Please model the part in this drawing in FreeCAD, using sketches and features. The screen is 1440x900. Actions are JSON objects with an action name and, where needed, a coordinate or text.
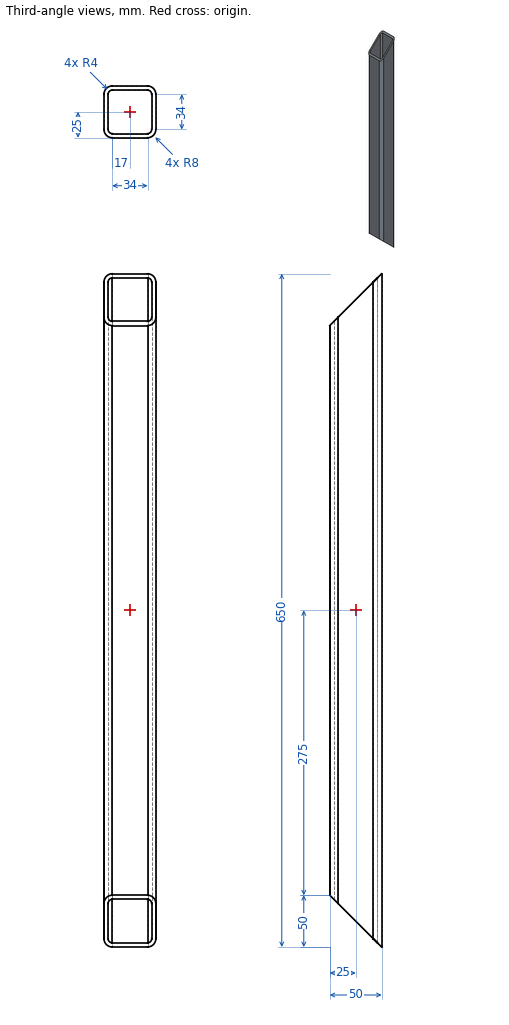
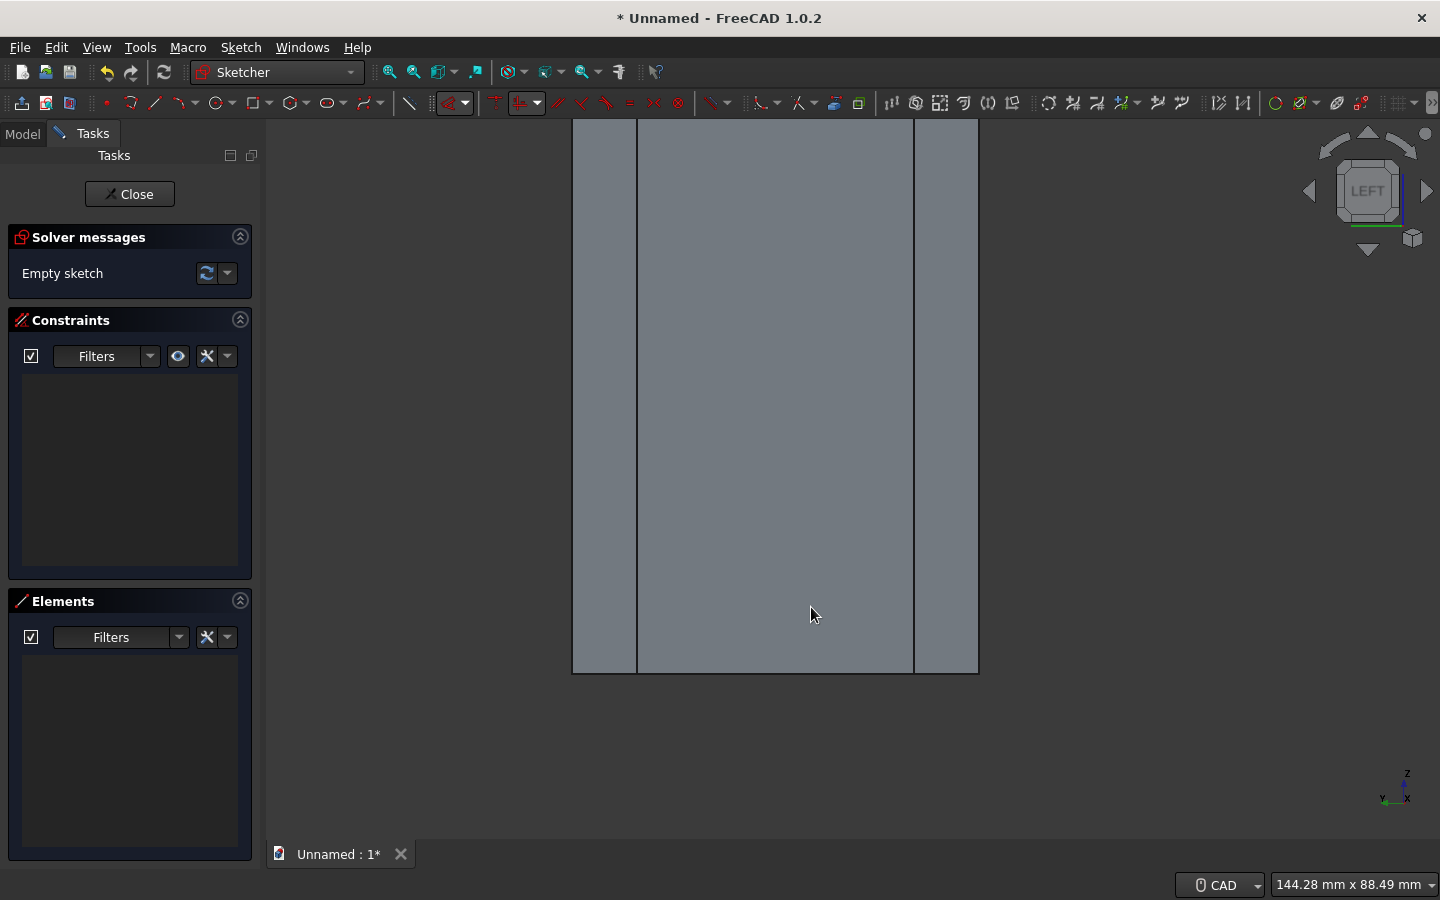
{"action": "left_click", "coordinate": [132, 104]}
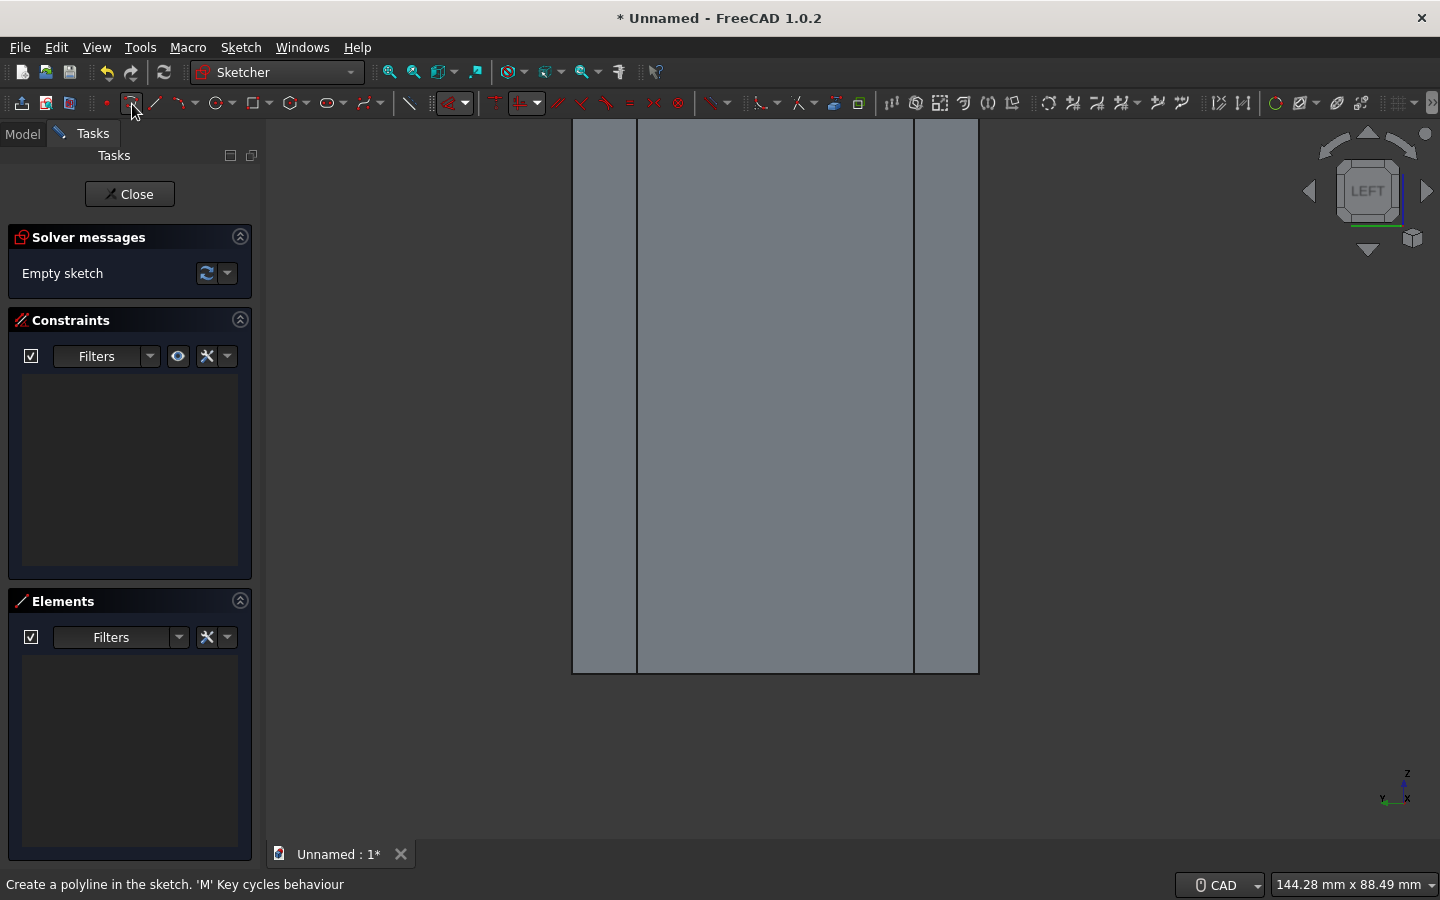
{"action": "left_click", "coordinate": [979, 267]}
{"action": "left_click", "coordinate": [572, 674]}
{"action": "left_click", "coordinate": [979, 674]}
{"action": "left_click", "coordinate": [979, 268]}
{"action": "key", "text": "Escape"}
{"action": "key", "text": "Escape"}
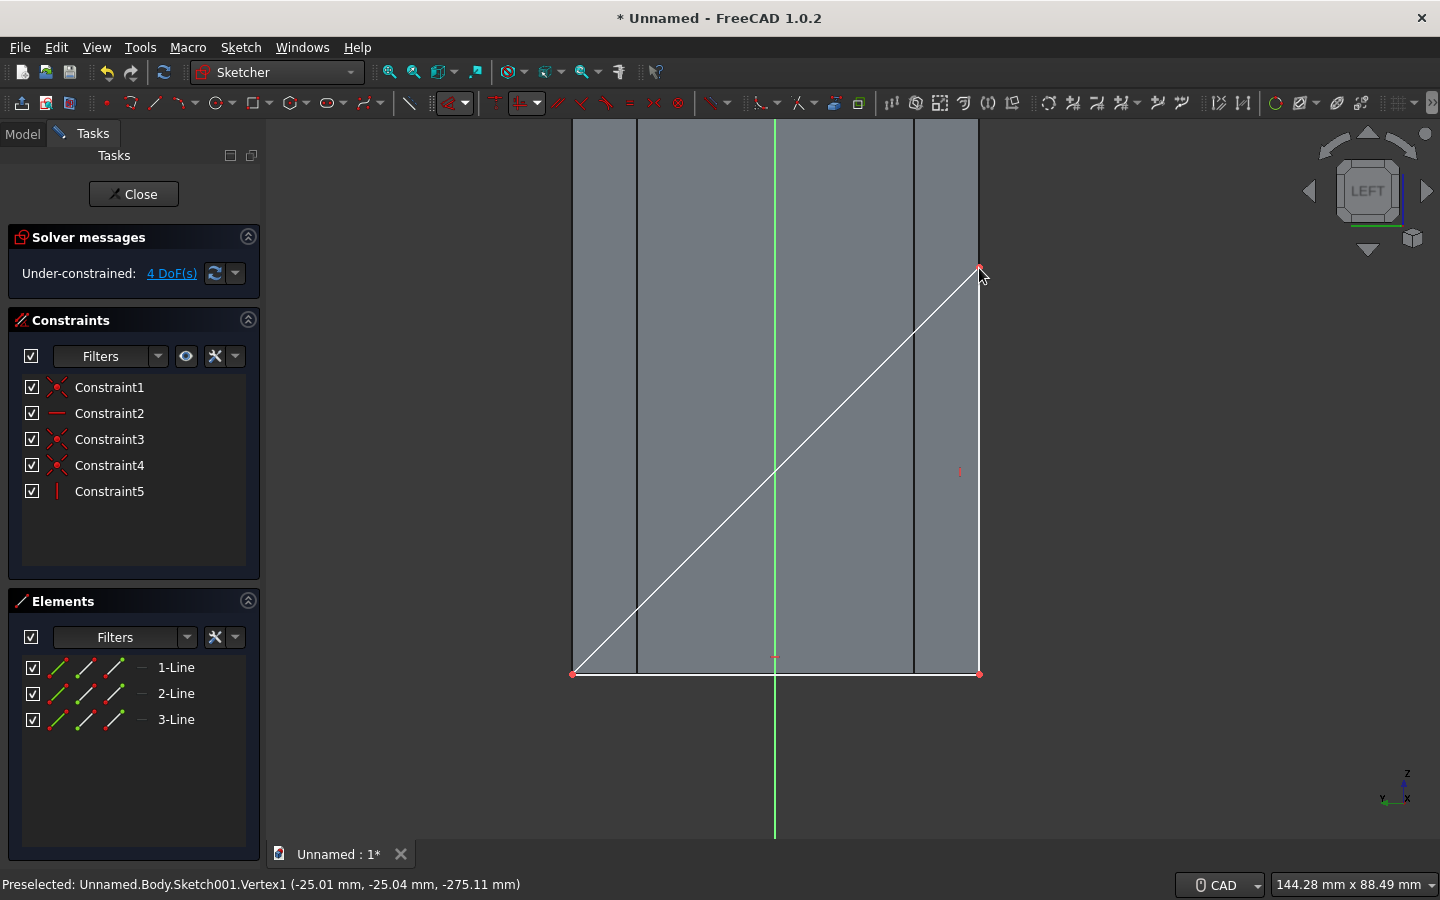
{"action": "left_click", "coordinate": [694, 675]}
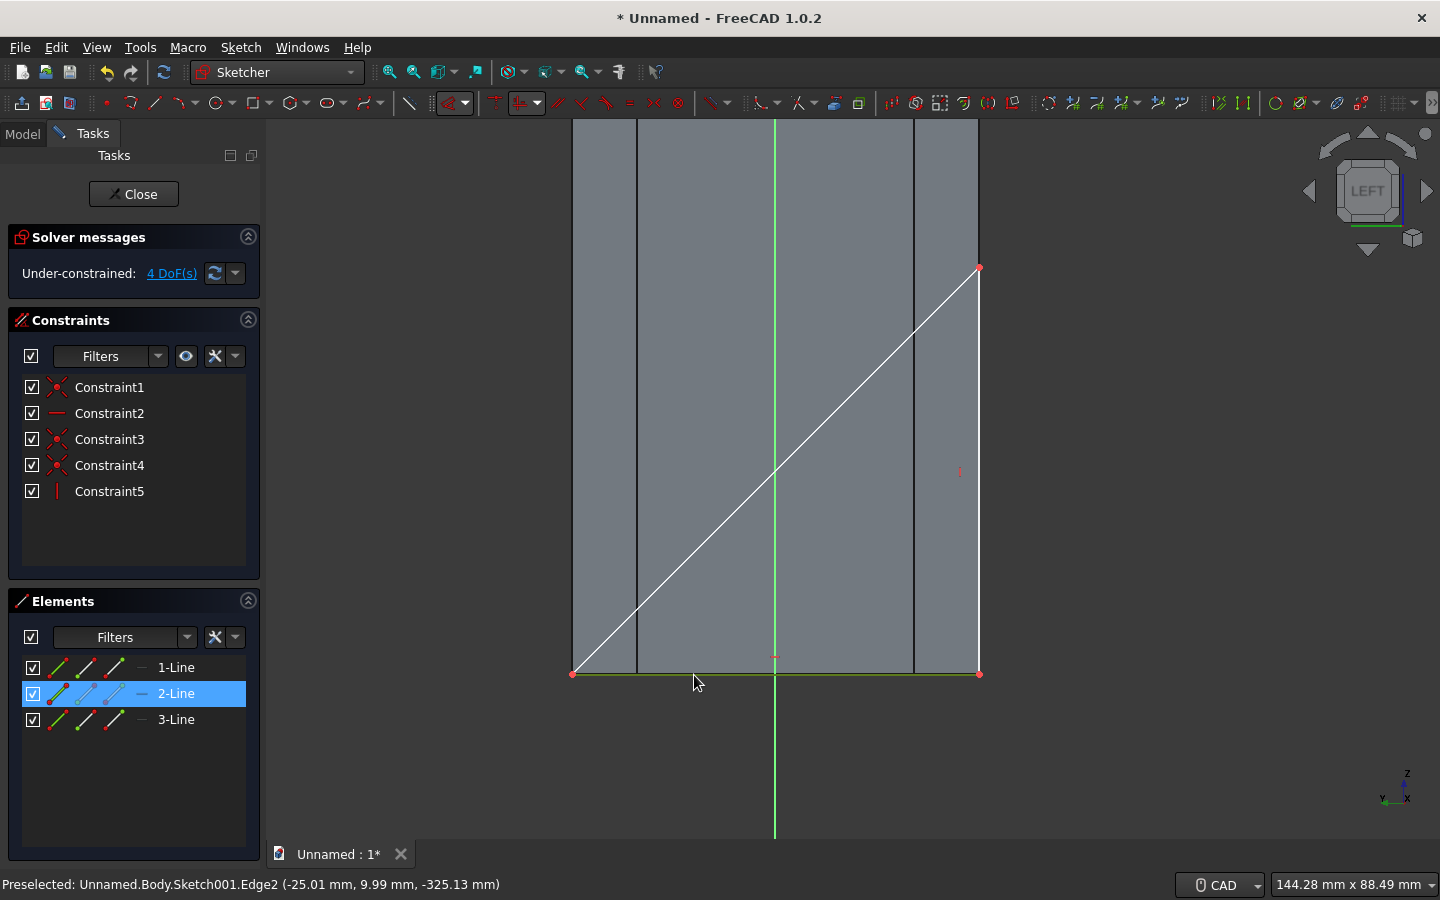
{"action": "left_click", "coordinate": [468, 104]}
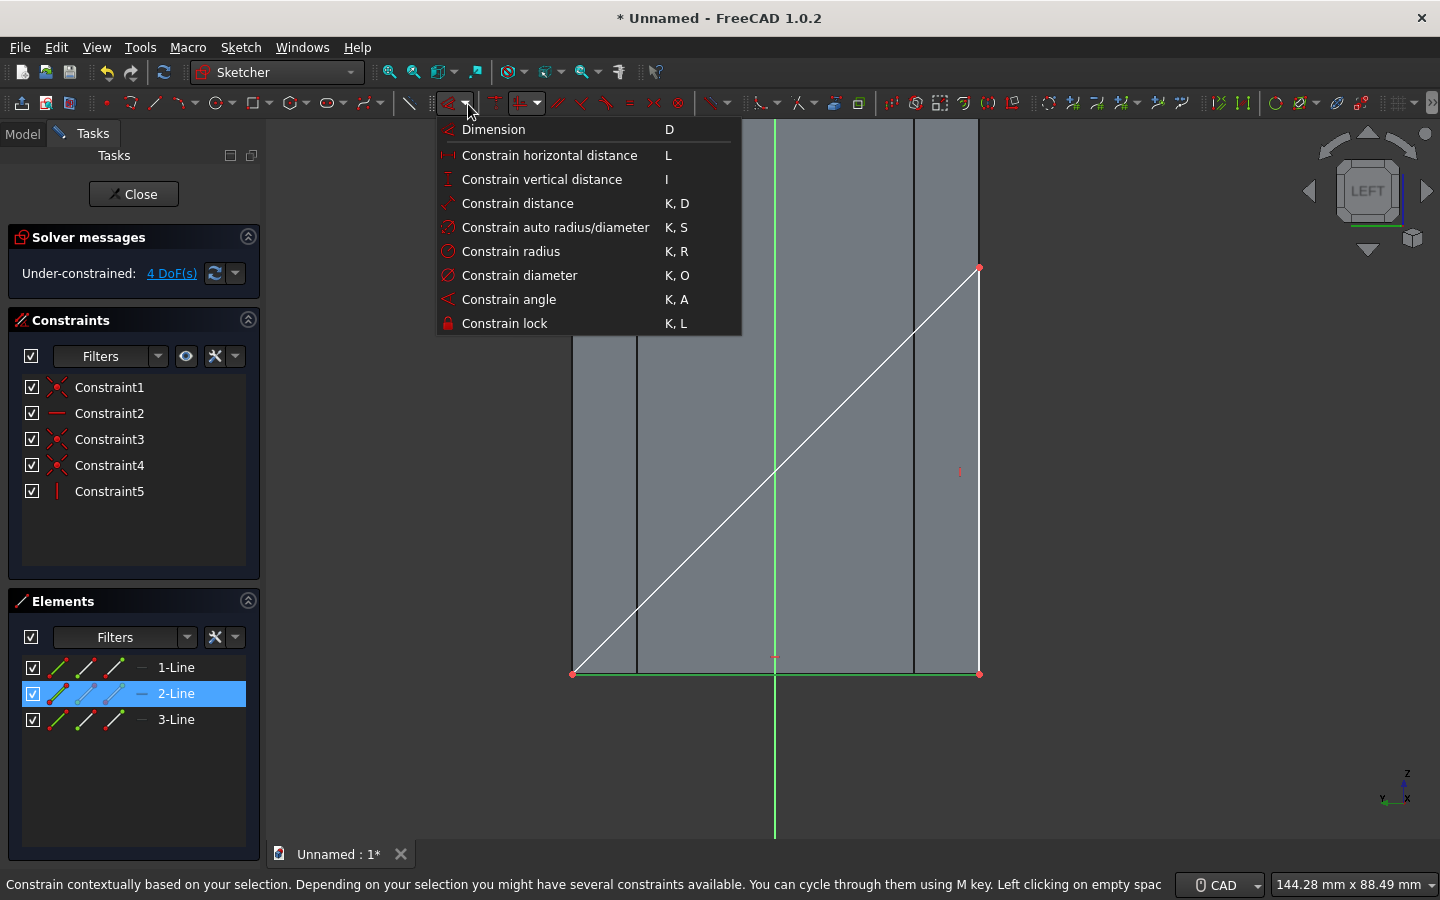
{"action": "left_click", "coordinate": [589, 155]}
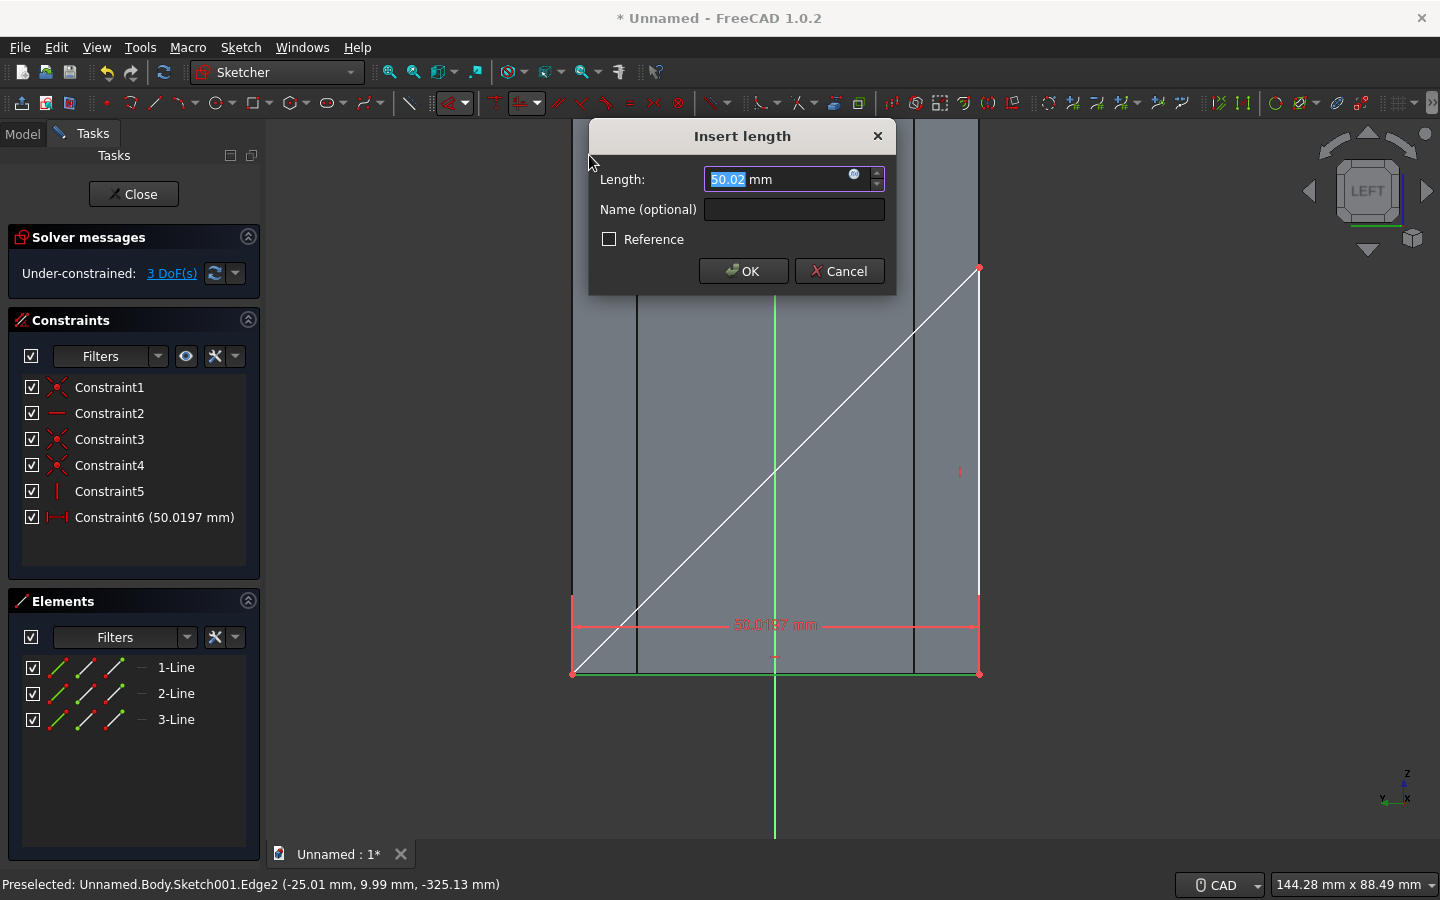
{"action": "type", "text": "50"}
{"action": "key", "text": "Return"}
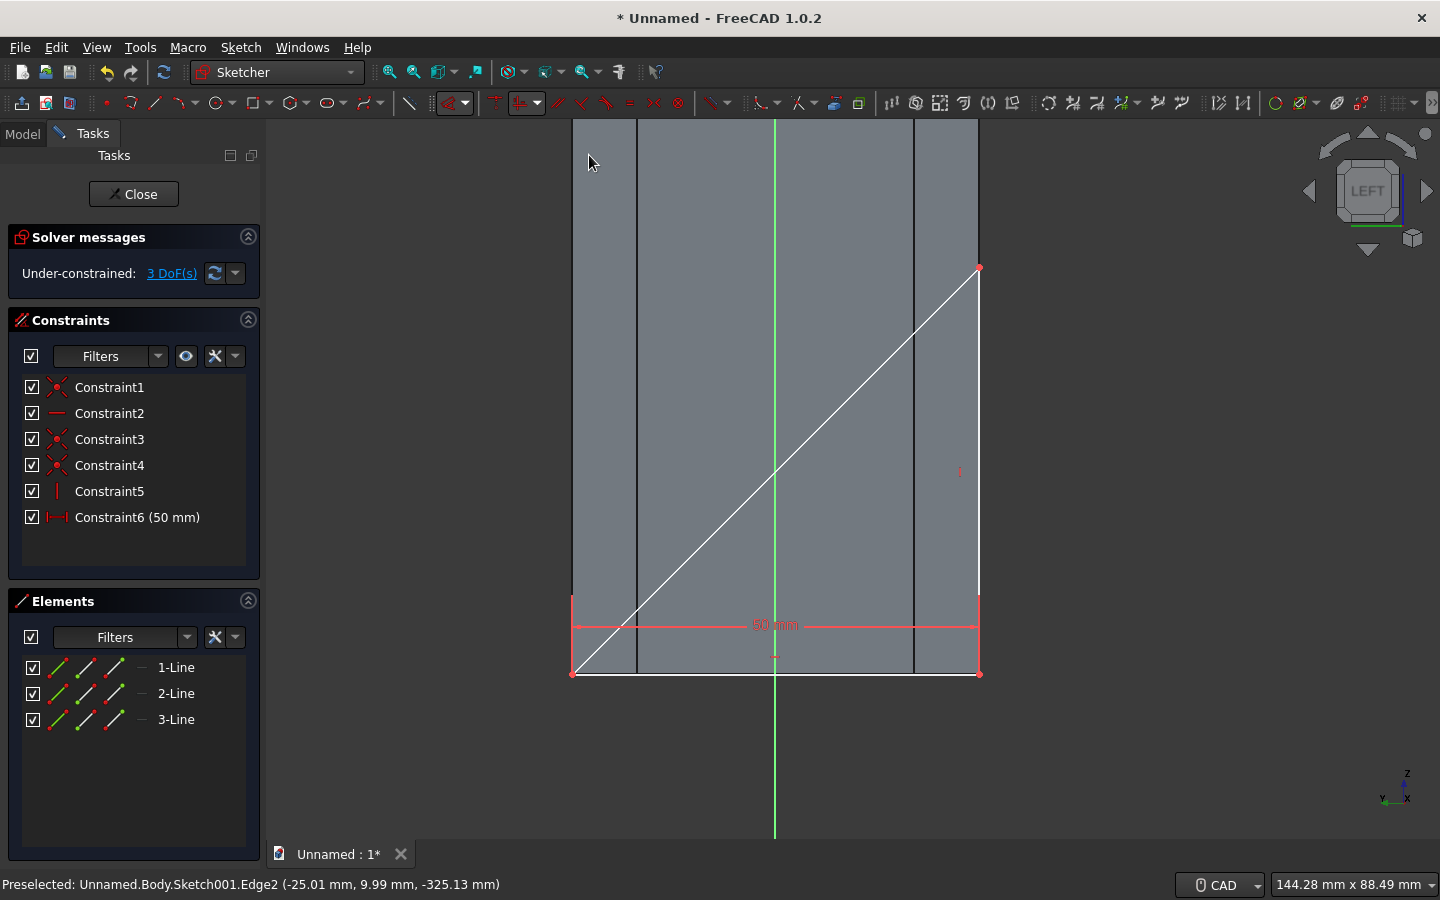
{"action": "left_click", "coordinate": [979, 553]}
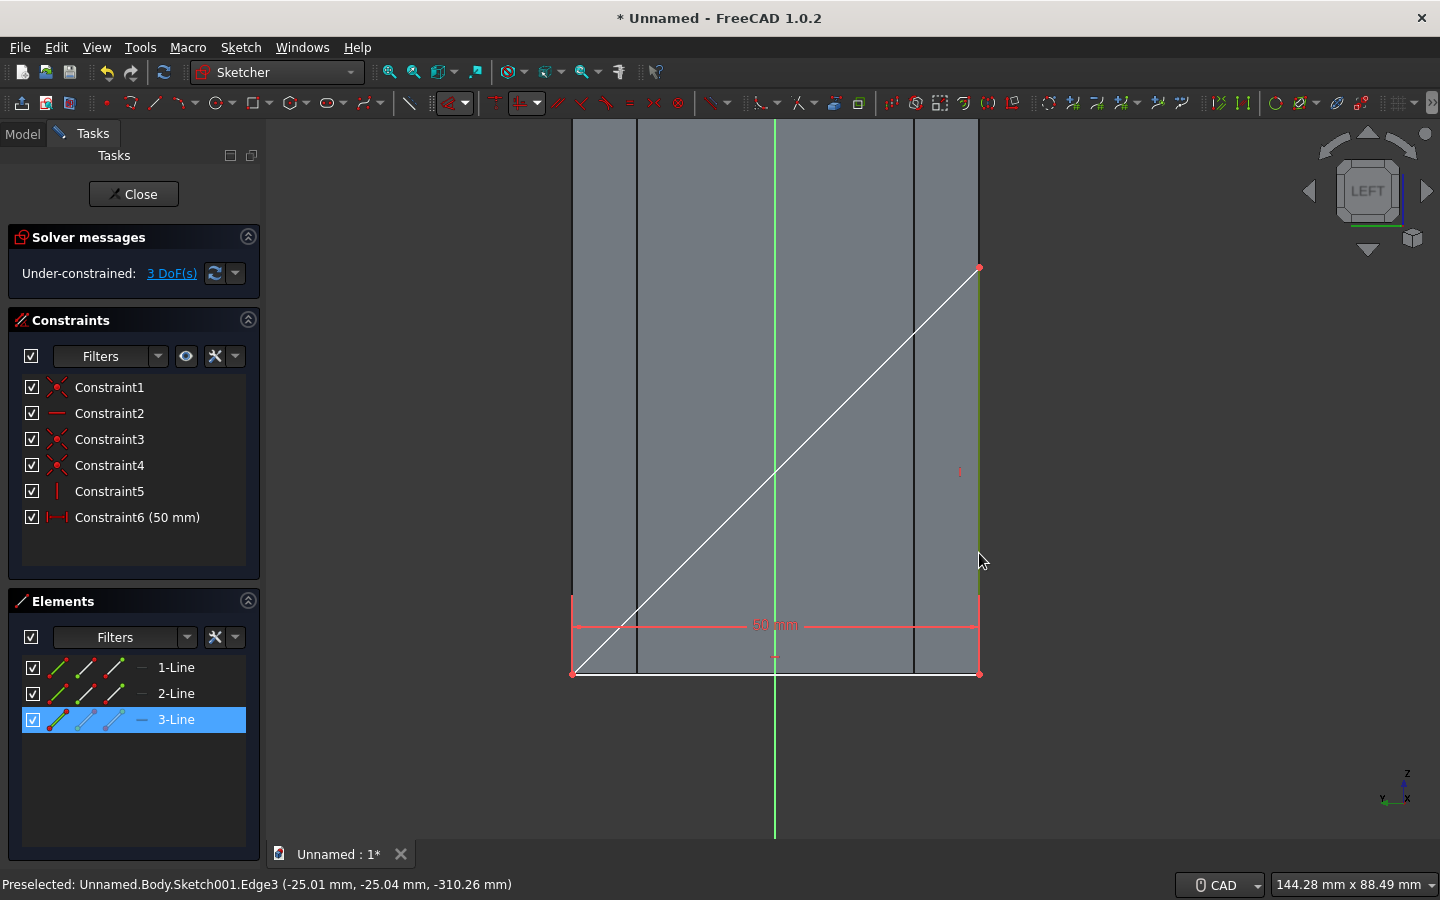
{"action": "key", "text": "i"}